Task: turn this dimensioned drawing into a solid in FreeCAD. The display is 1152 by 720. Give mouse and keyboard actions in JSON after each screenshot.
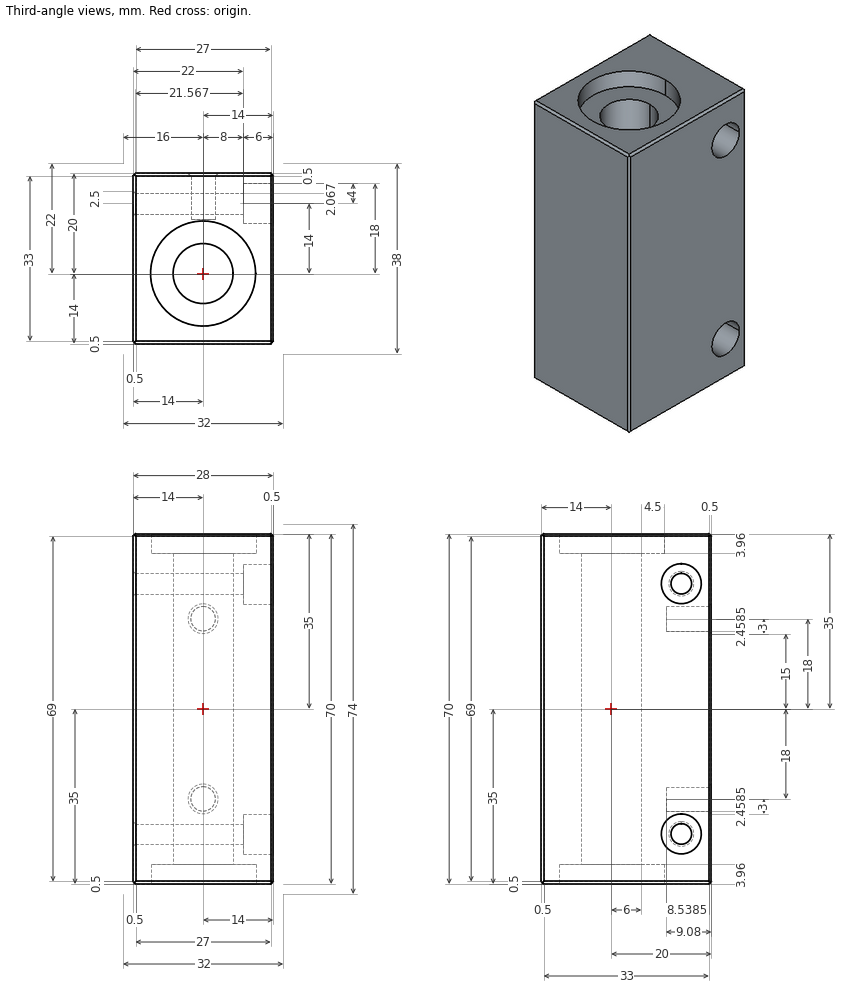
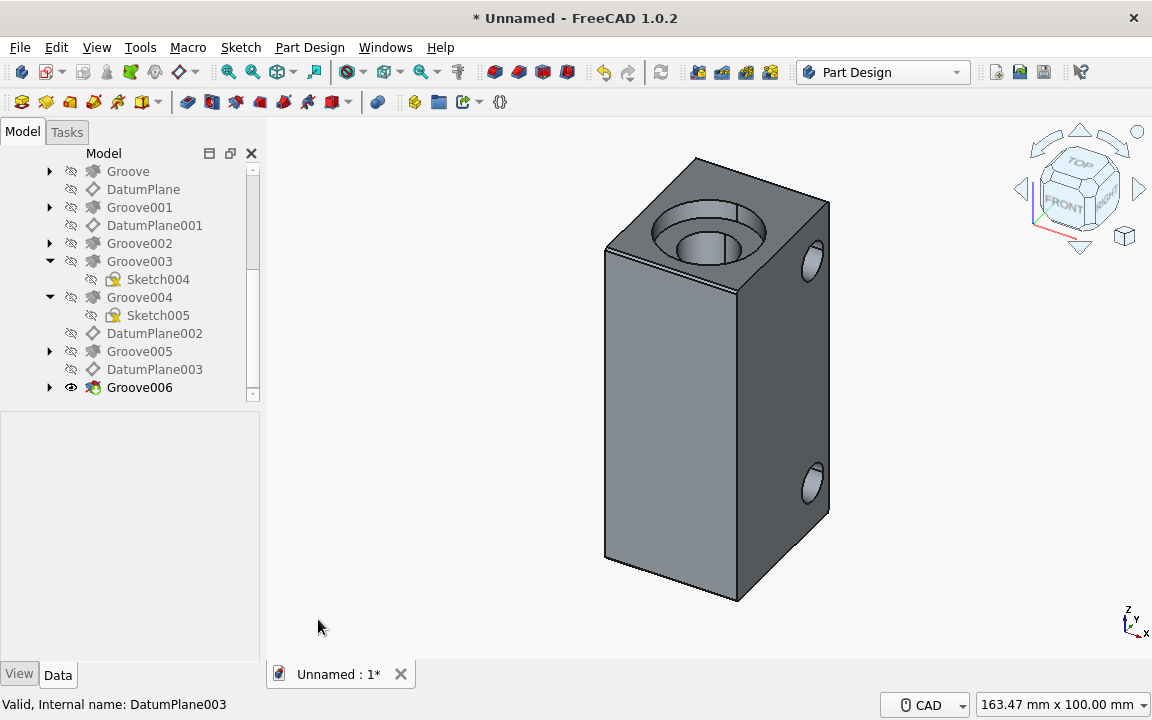
{"action": "left_click", "coordinate": [46, 72]}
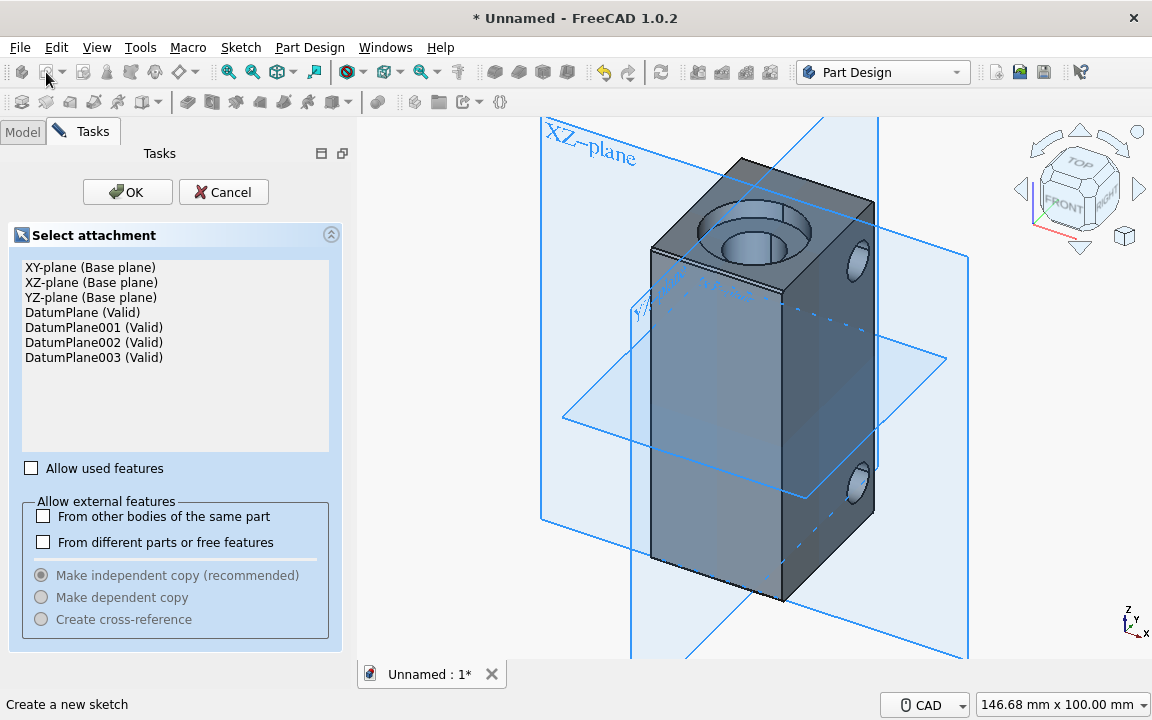
{"action": "left_click", "coordinate": [82, 268]}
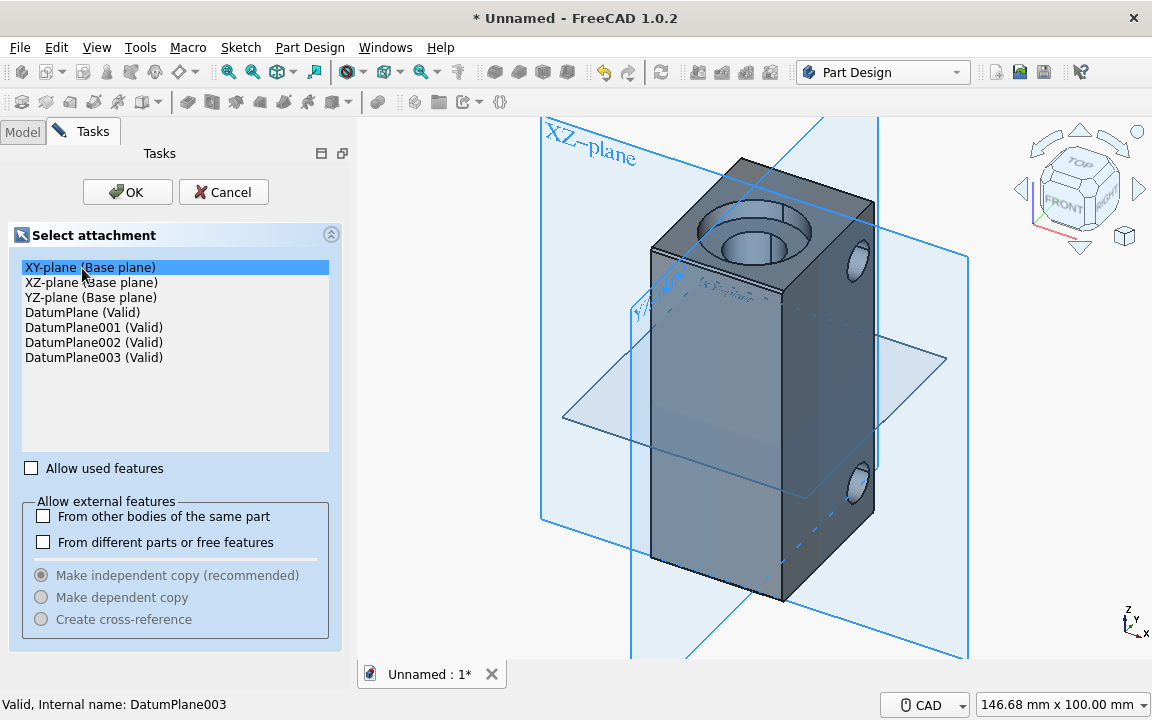
{"action": "left_click", "coordinate": [128, 192]}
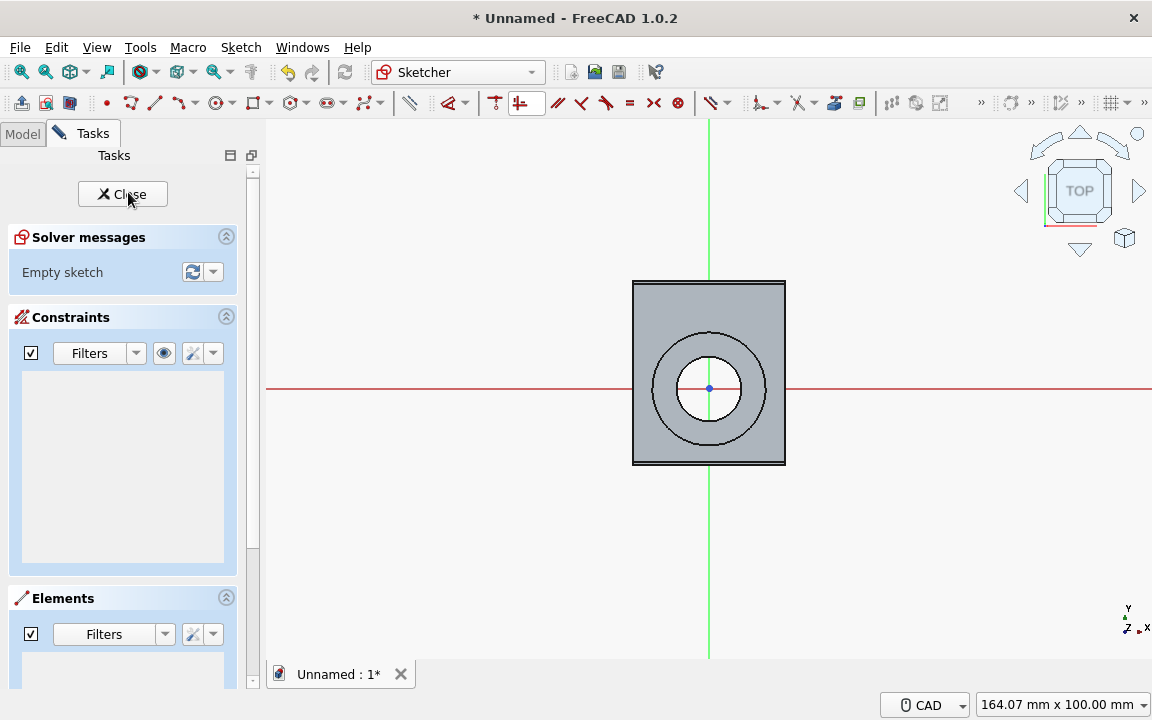
{"action": "left_click", "coordinate": [70, 104]}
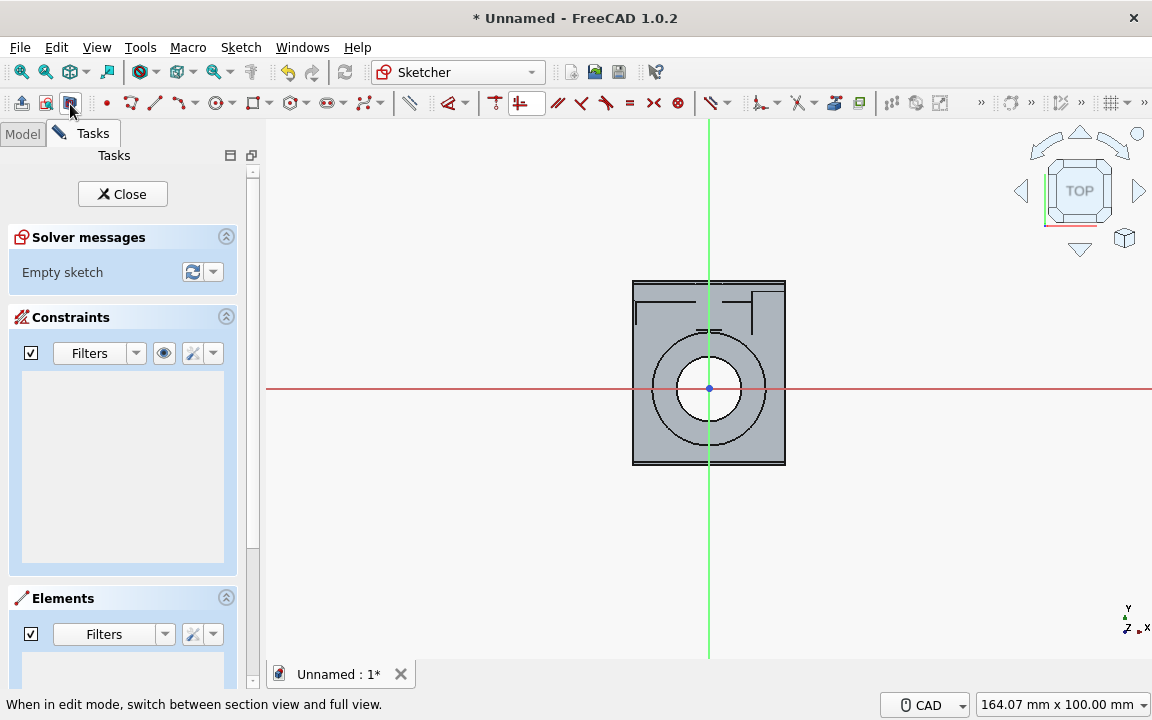
{"action": "scroll", "coordinate": [792, 353], "scroll_direction": "up", "scroll_amount": 3}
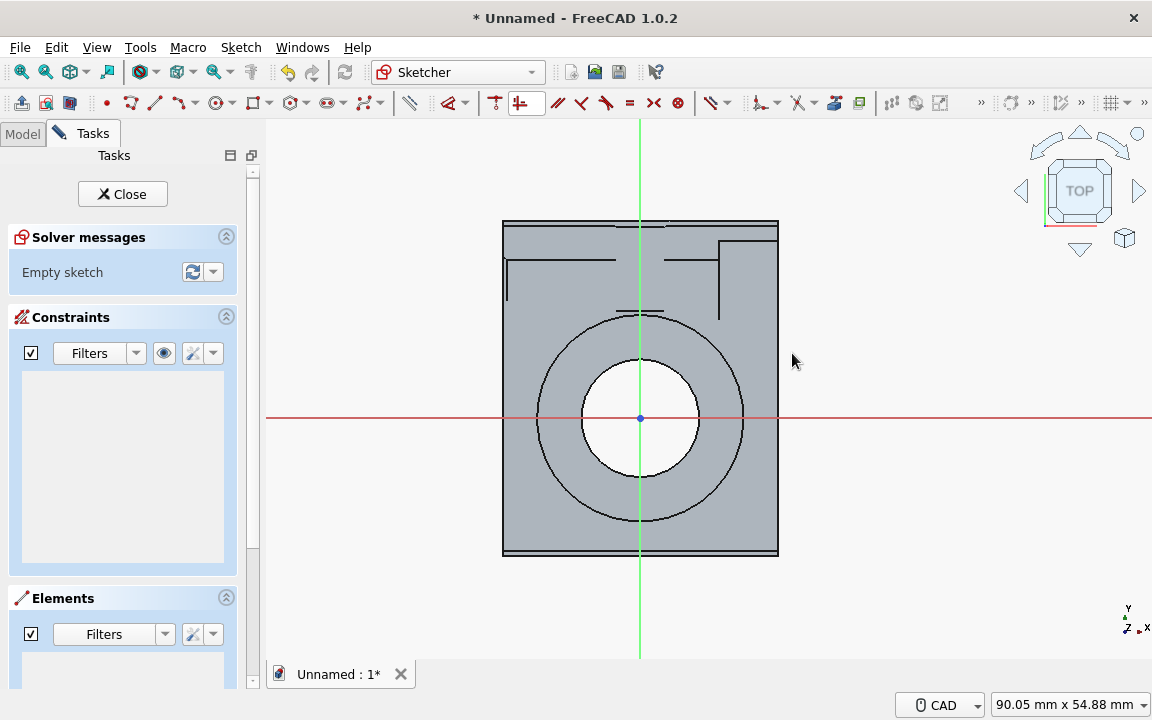
{"action": "left_click", "coordinate": [254, 104]}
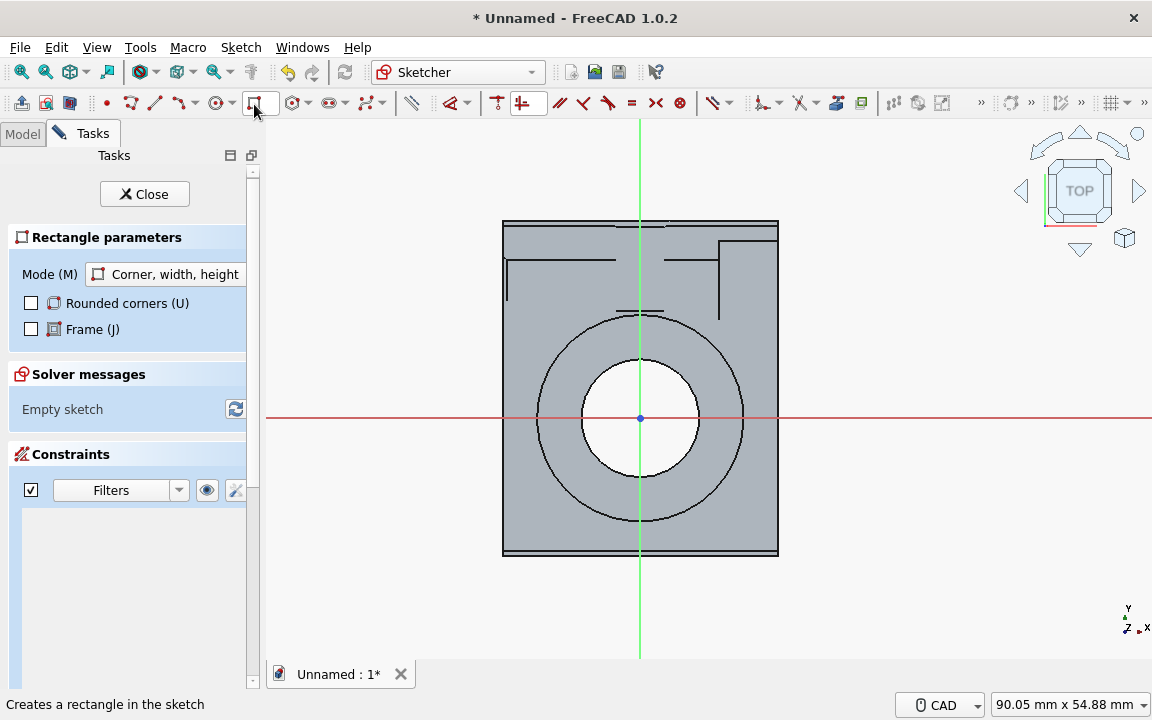
{"action": "left_click", "coordinate": [483, 202]}
{"action": "mouse_move", "coordinate": [798, 576]}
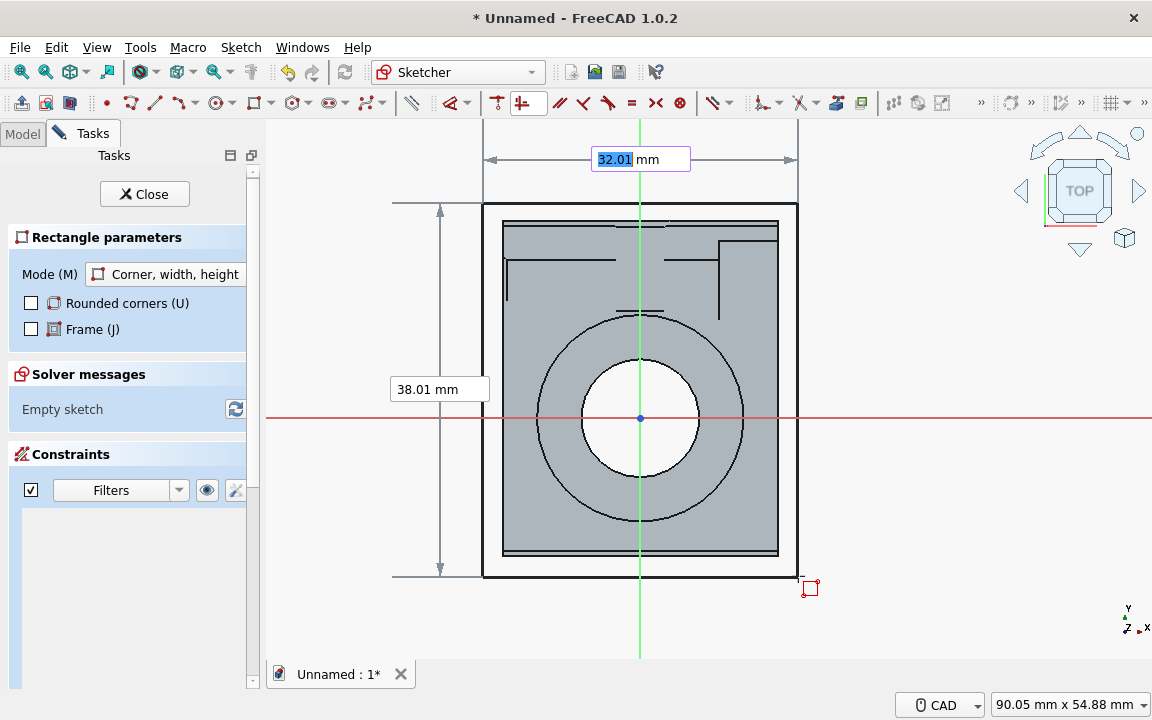
{"action": "type", "text": "32"}
{"action": "key", "text": "Tab"}
{"action": "type", "text": "38"}
{"action": "key", "text": "Return"}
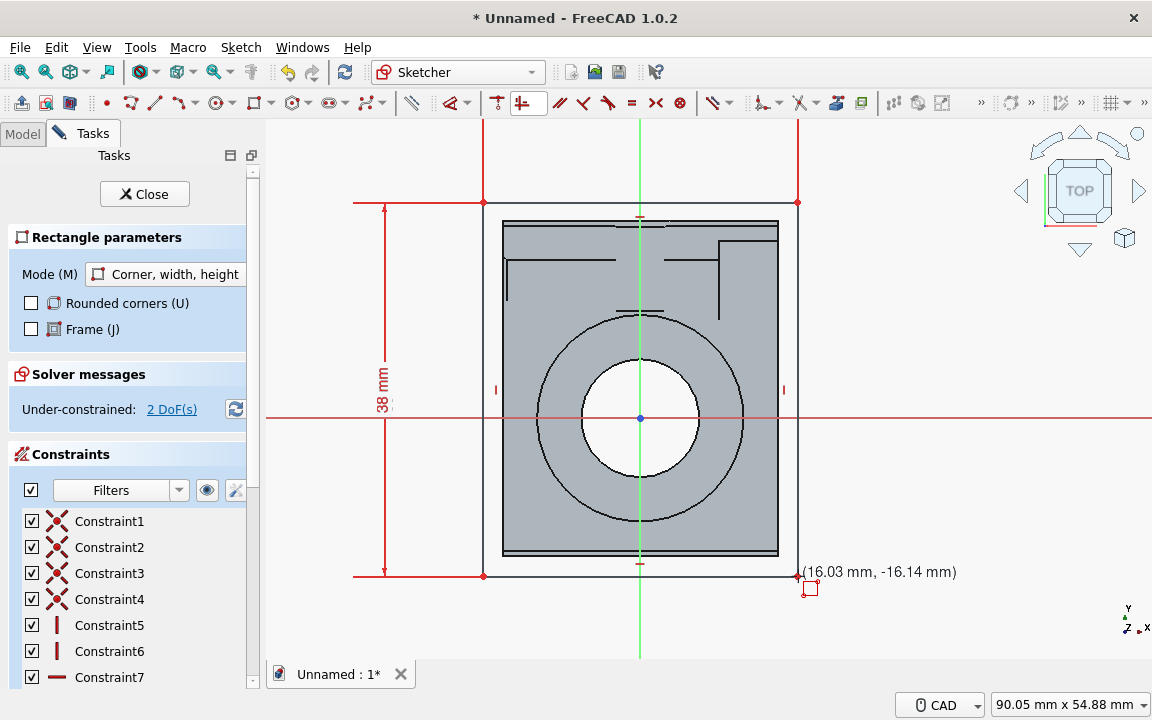
{"action": "left_click", "coordinate": [132, 104]}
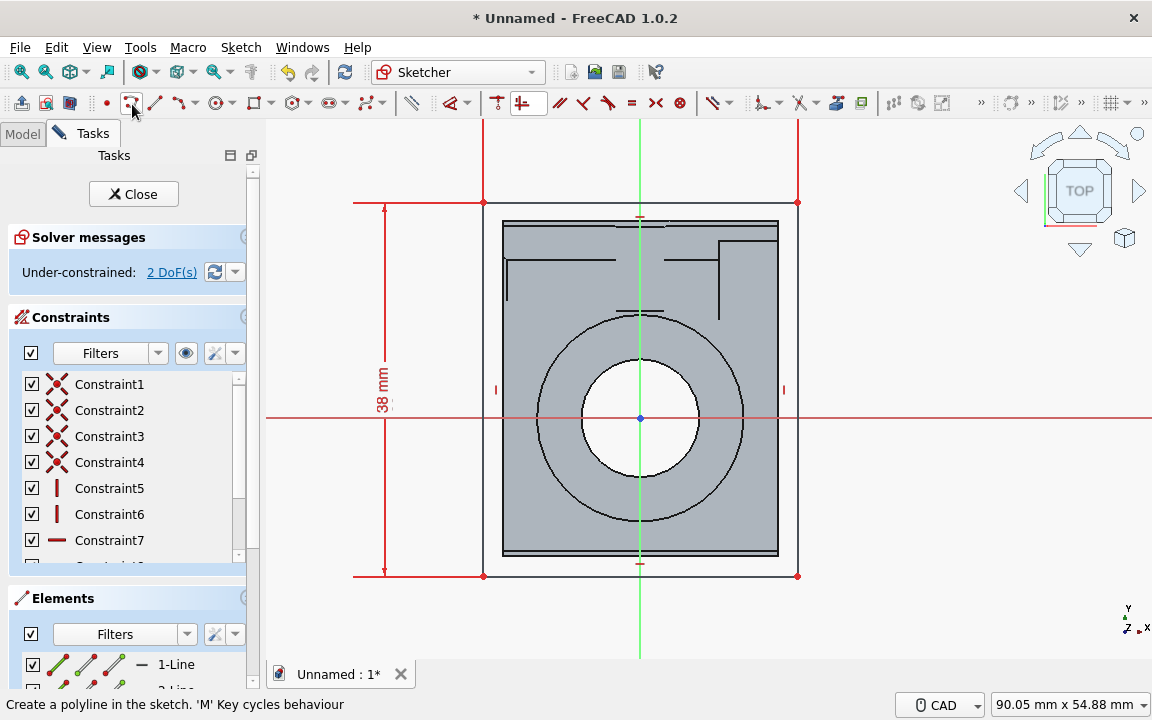
{"action": "left_click", "coordinate": [507, 556]}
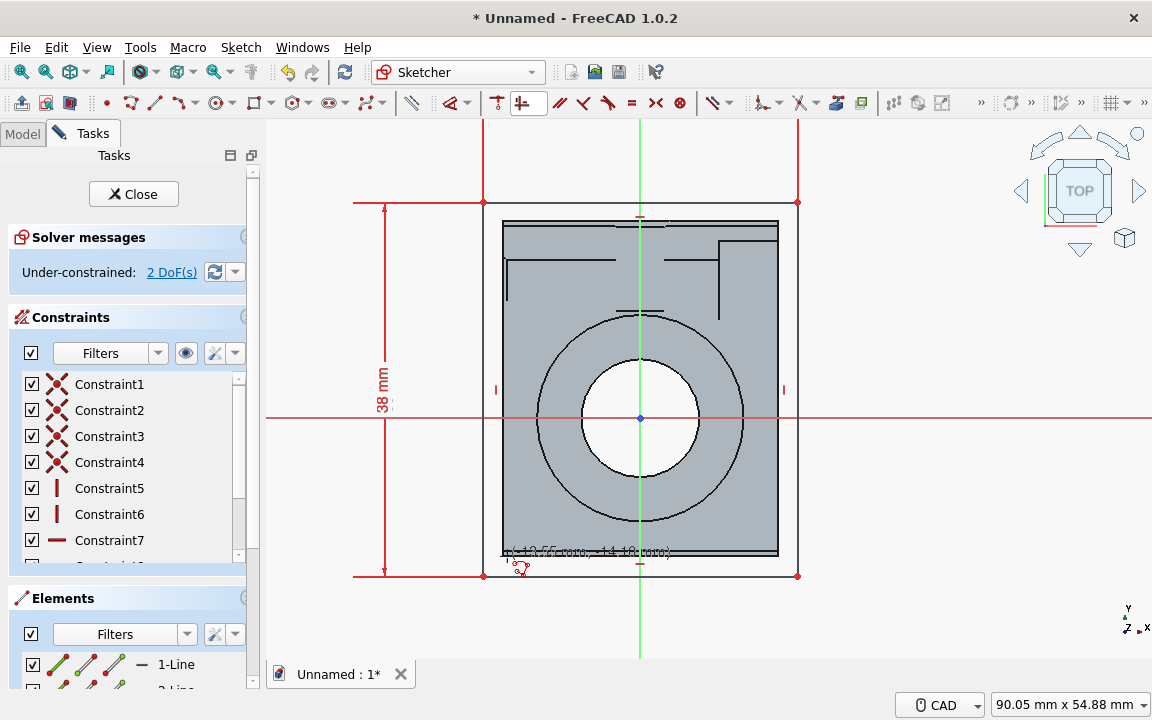
{"action": "scroll", "coordinate": [503, 551], "scroll_direction": "up", "scroll_amount": 5}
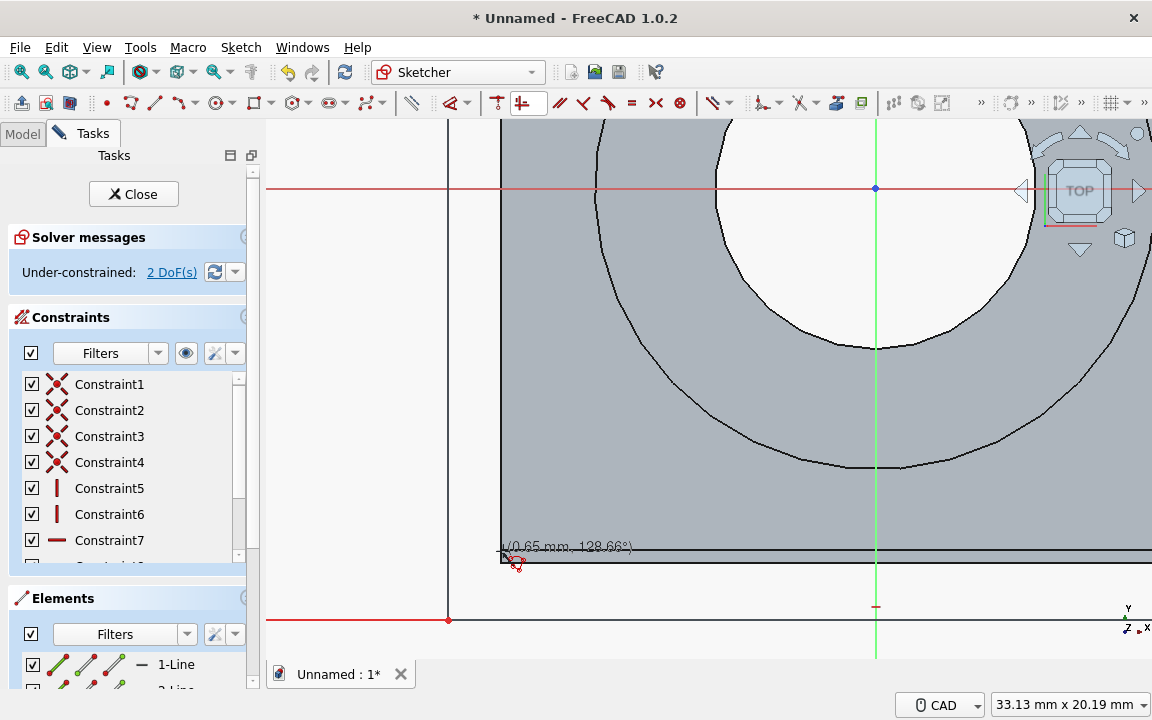
{"action": "left_click", "coordinate": [501, 550]}